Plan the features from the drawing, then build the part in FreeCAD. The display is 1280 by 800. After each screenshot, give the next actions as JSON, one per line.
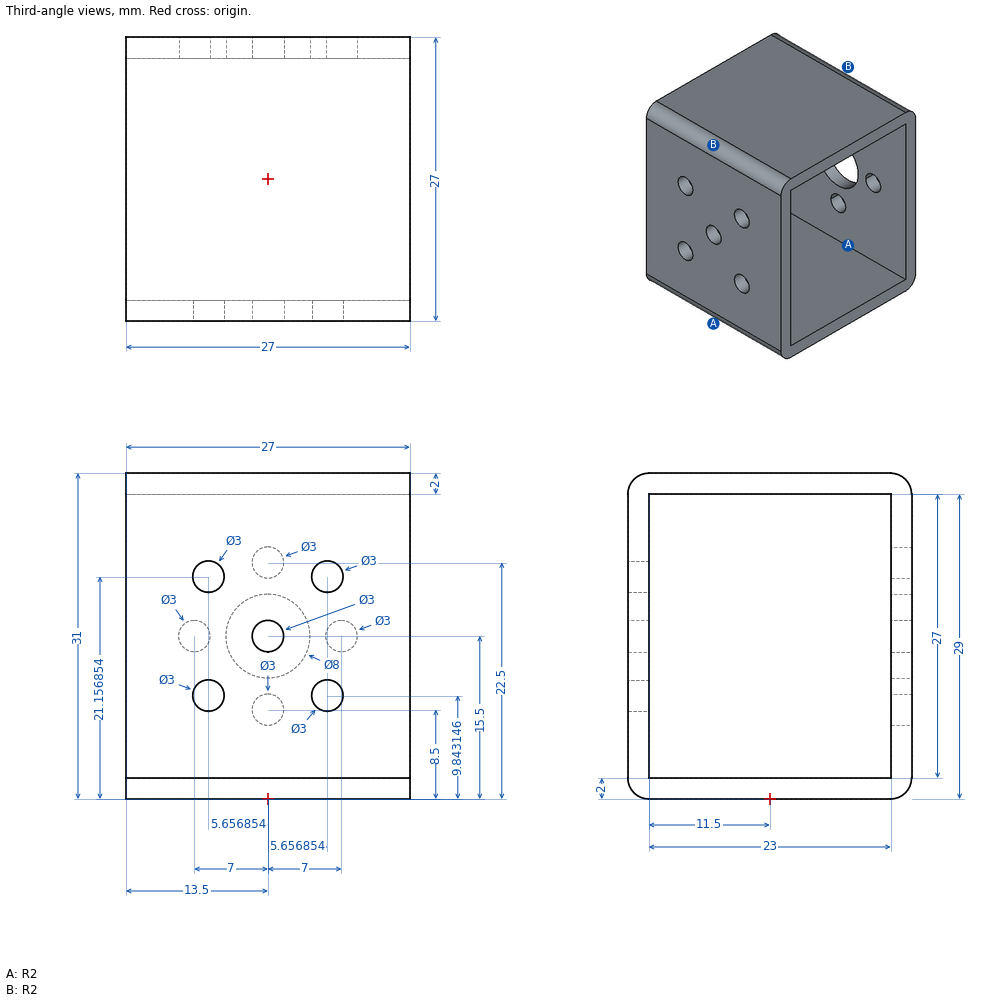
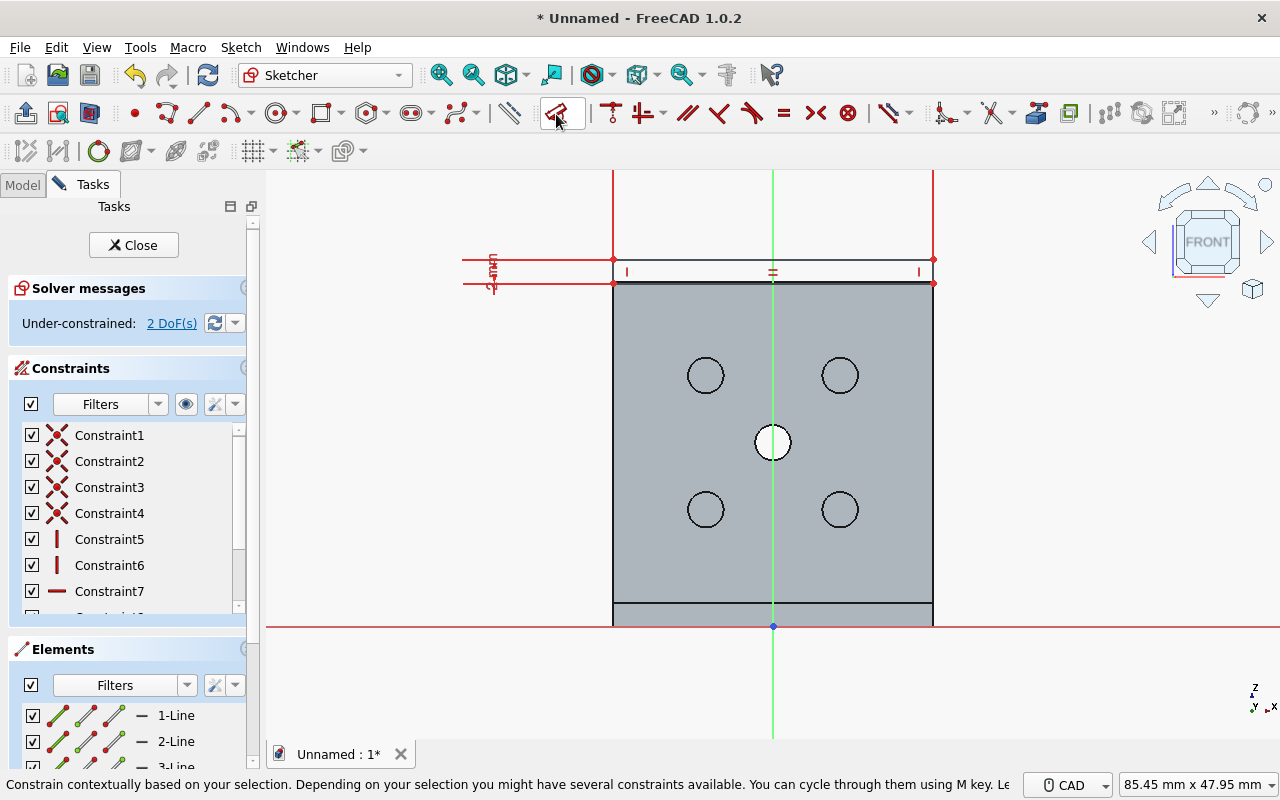
{"action": "left_click", "coordinate": [613, 260]}
{"action": "left_click", "coordinate": [579, 443]}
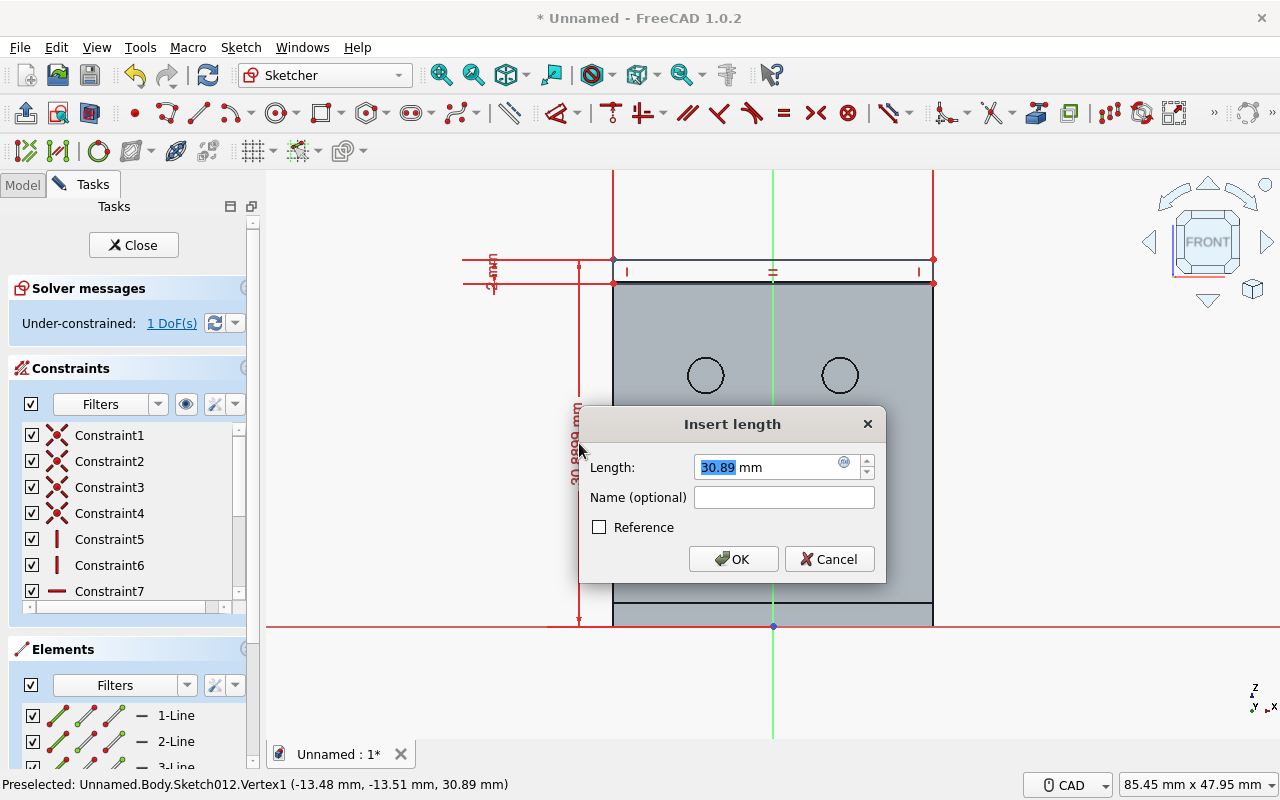
{"action": "type", "text": "31"}
{"action": "key", "text": "Return"}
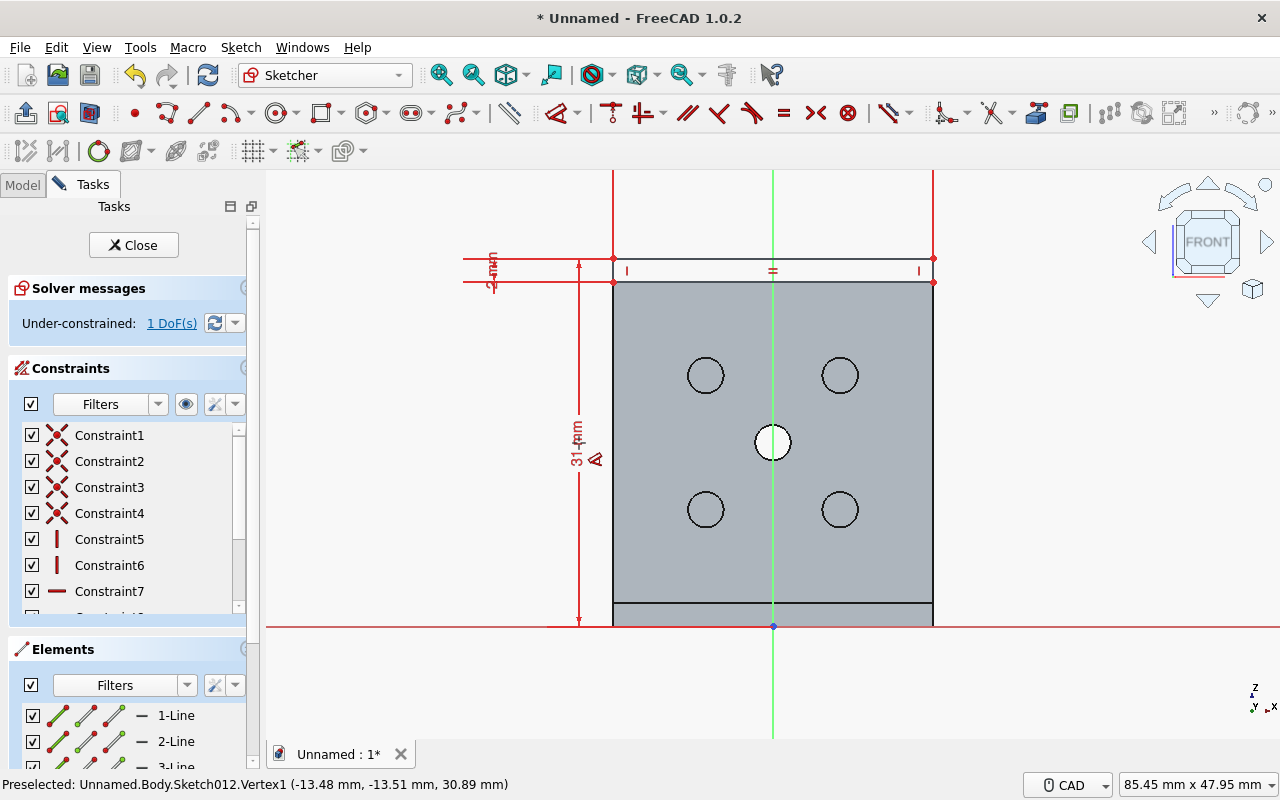
{"action": "left_click", "coordinate": [613, 259]}
{"action": "left_click", "coordinate": [693, 661]}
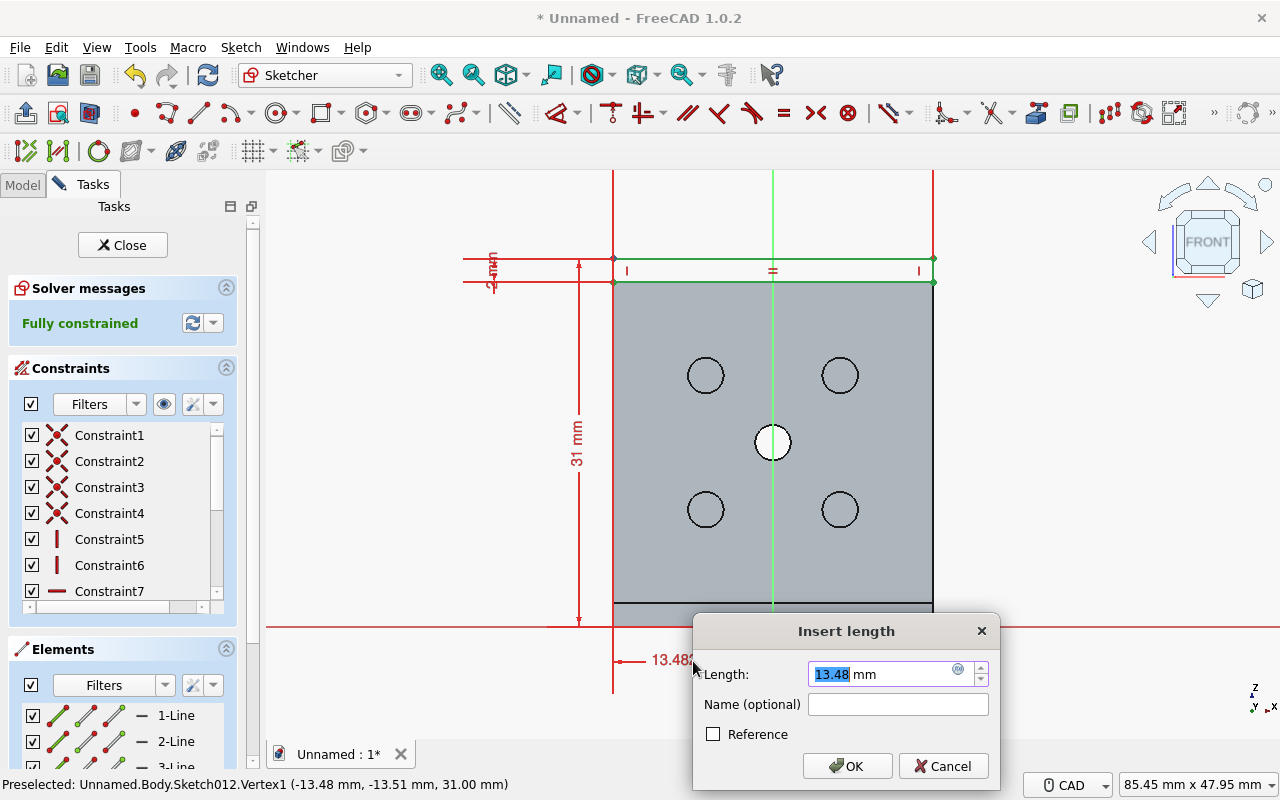
{"action": "type", "text": "13.5"}
{"action": "key", "text": "Return"}
{"action": "key", "text": "Escape"}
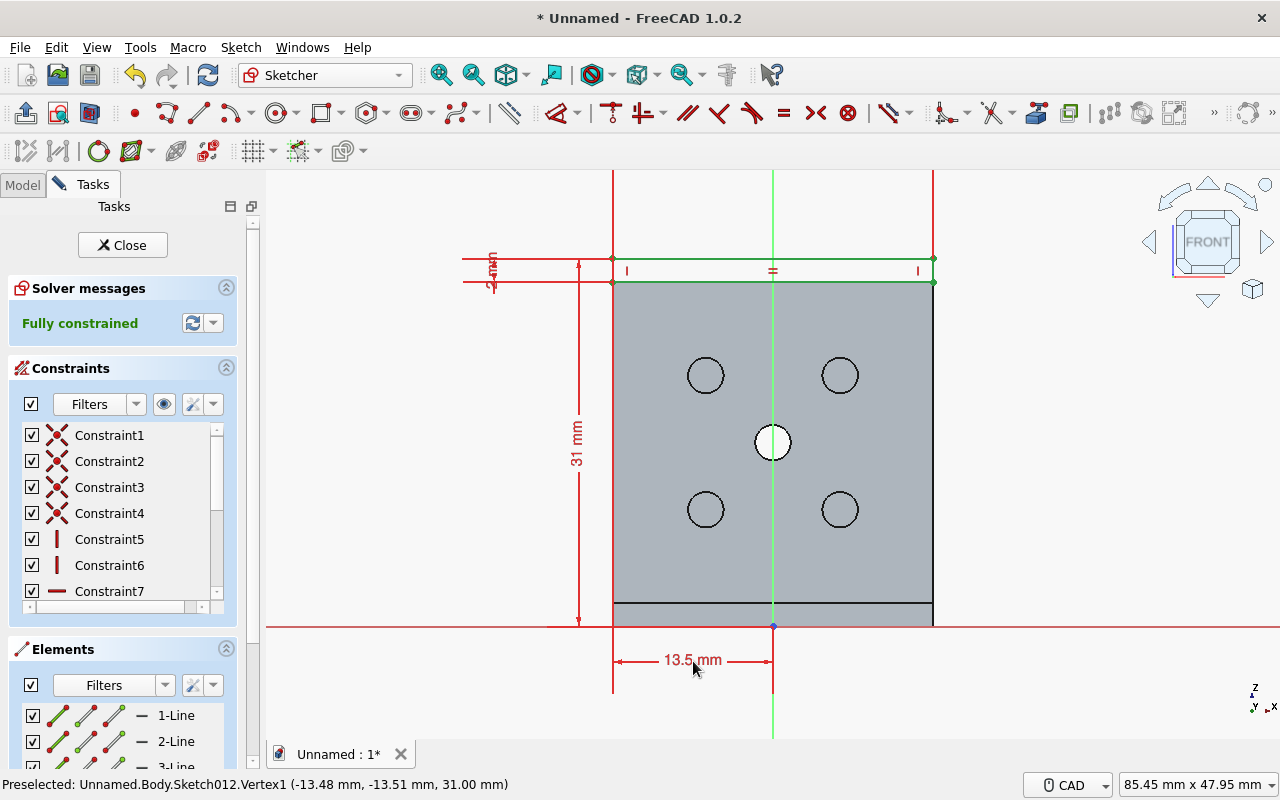
{"action": "left_click", "coordinate": [123, 245]}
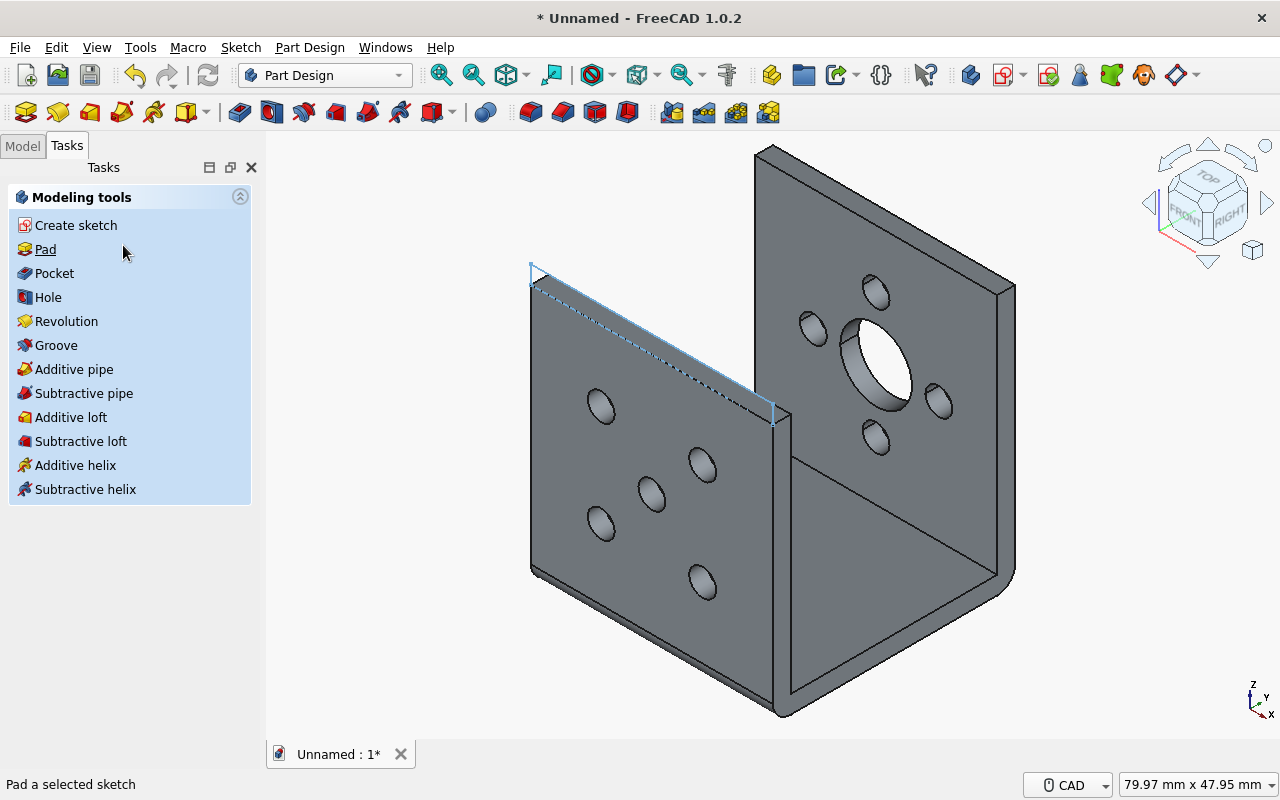
{"action": "left_click", "coordinate": [26, 112]}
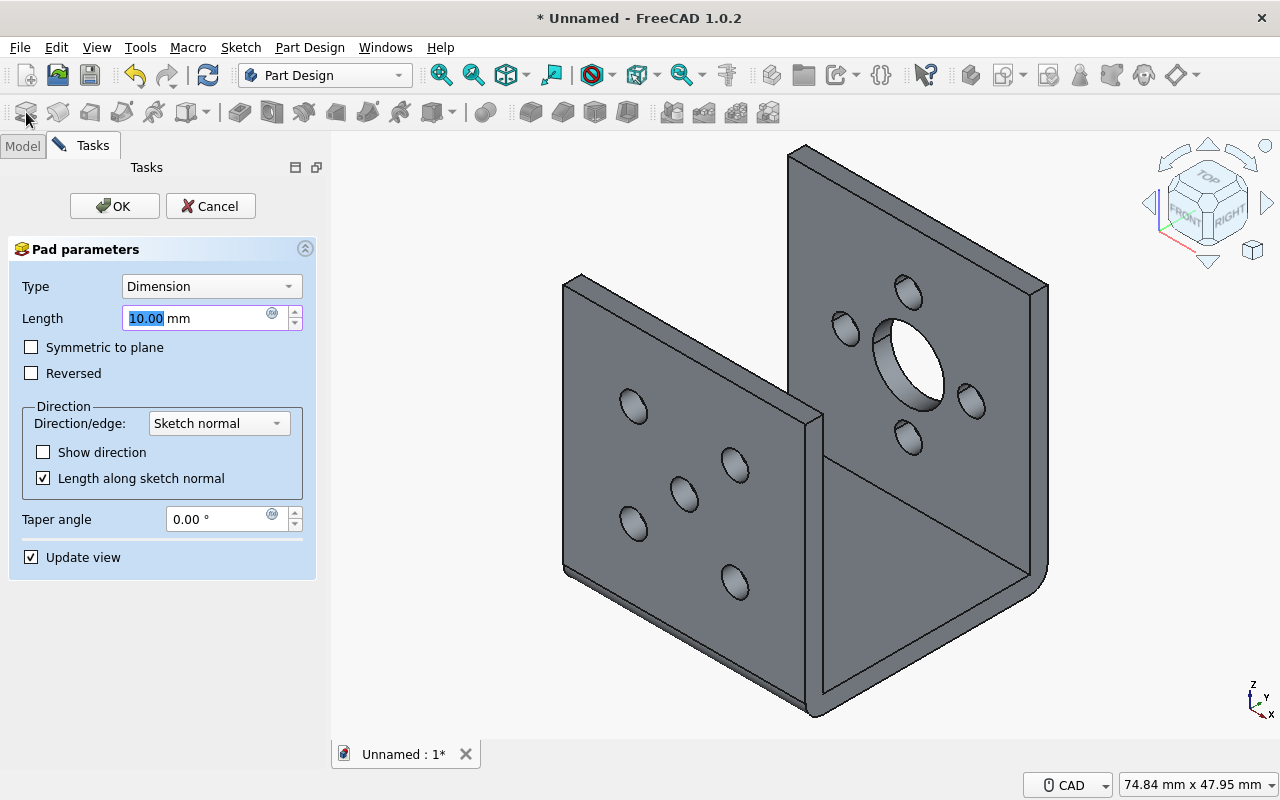
{"action": "type", "text": "27"}
{"action": "key", "text": "Tab"}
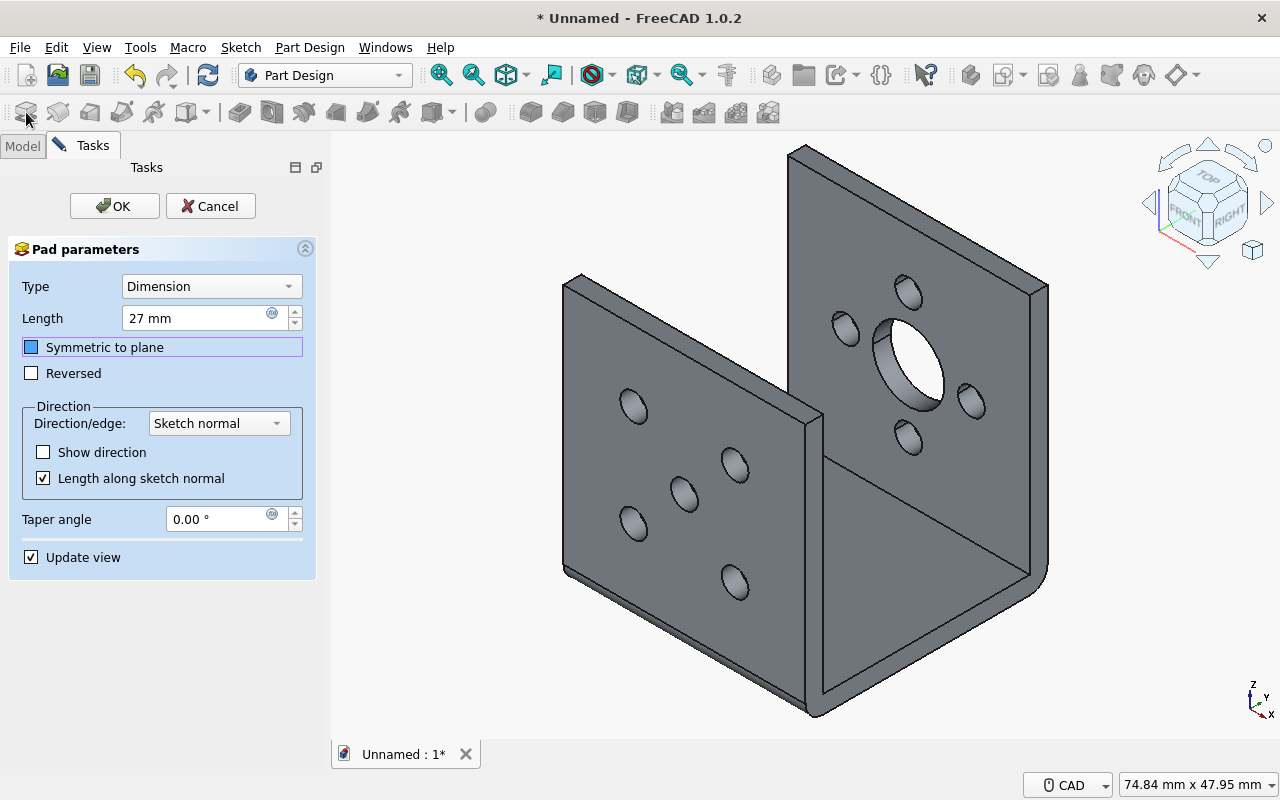
{"action": "left_click", "coordinate": [30, 373]}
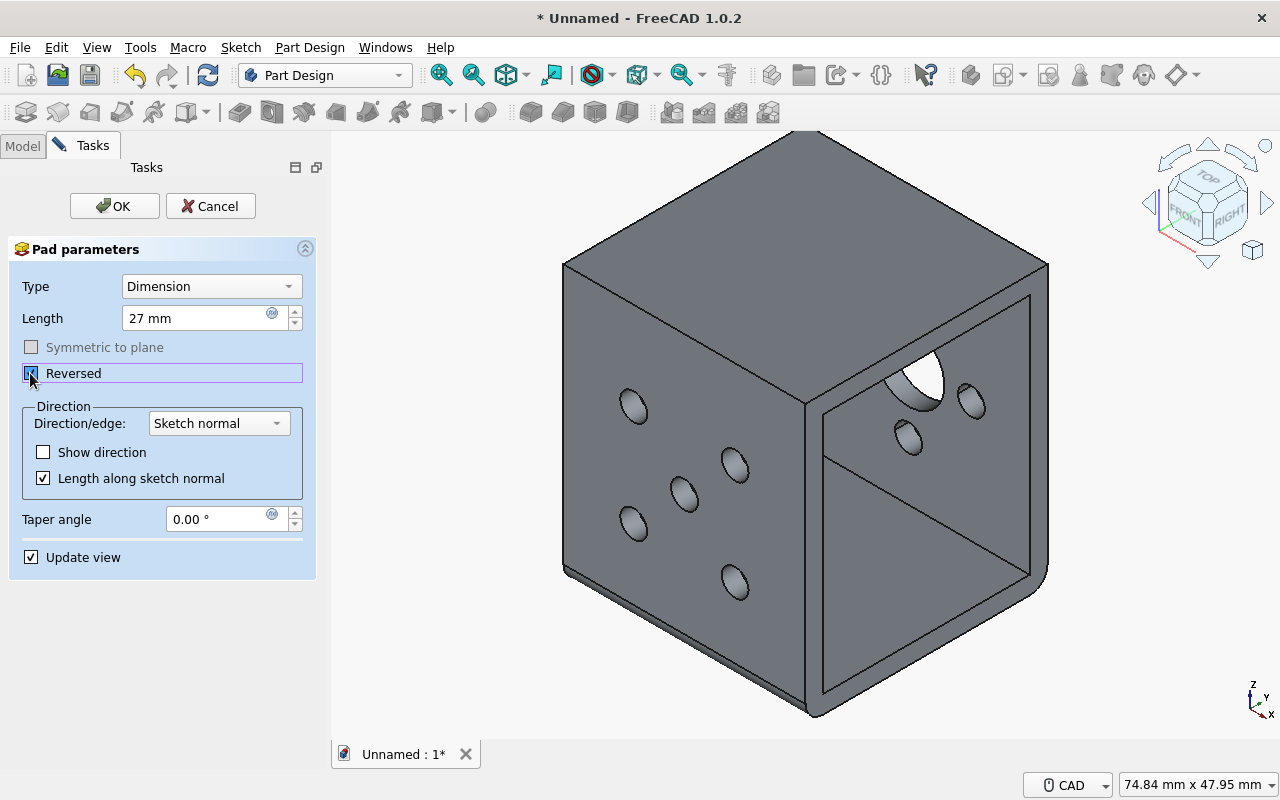
{"action": "left_click", "coordinate": [115, 206]}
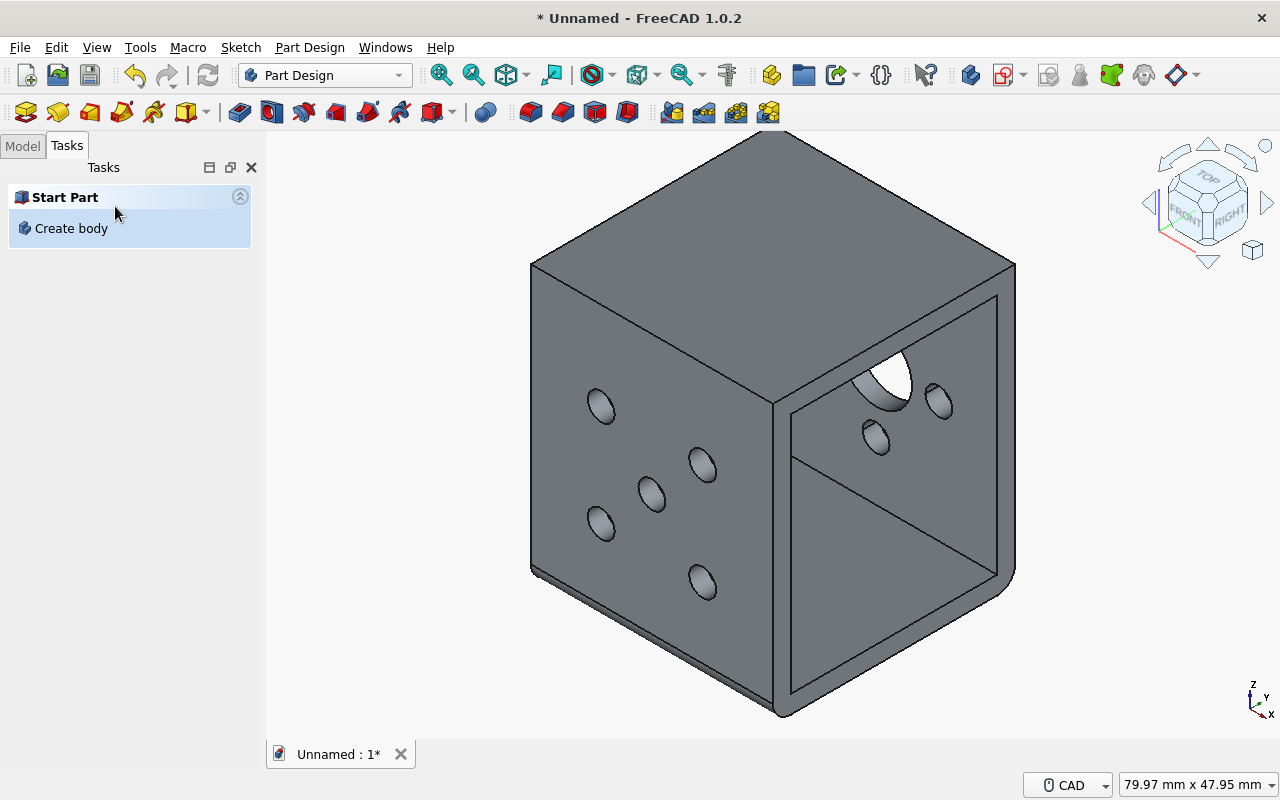
{"action": "key", "text": "v f"}